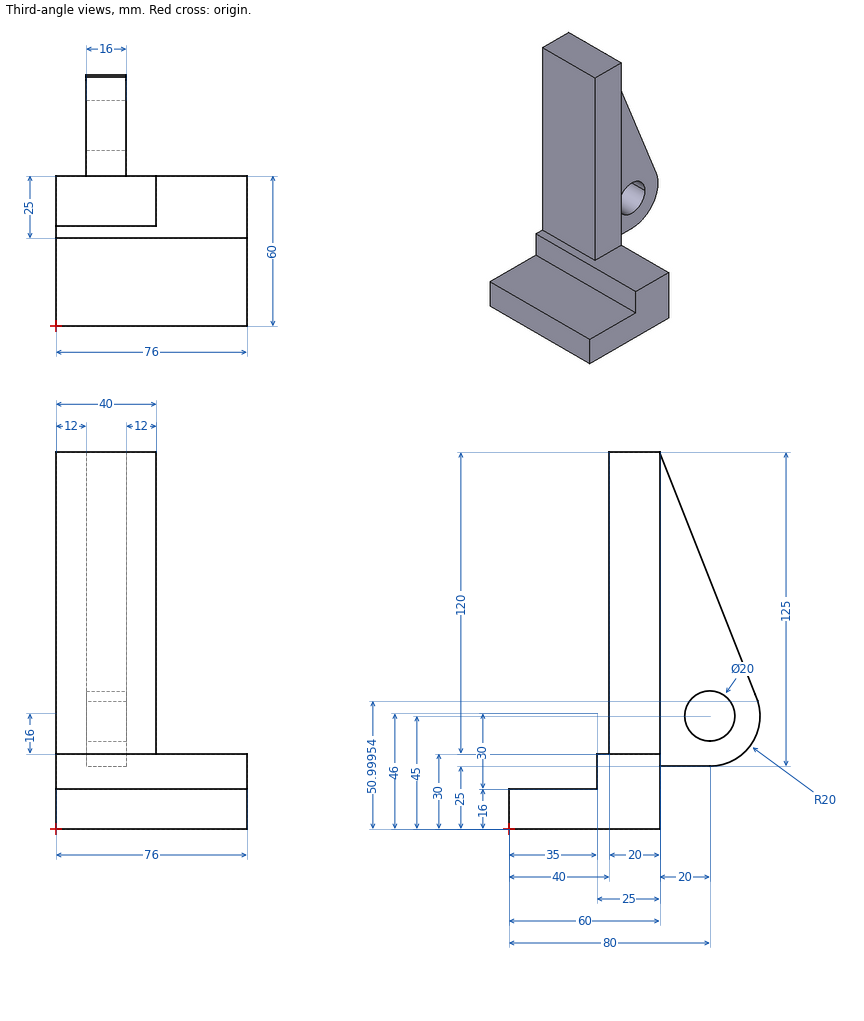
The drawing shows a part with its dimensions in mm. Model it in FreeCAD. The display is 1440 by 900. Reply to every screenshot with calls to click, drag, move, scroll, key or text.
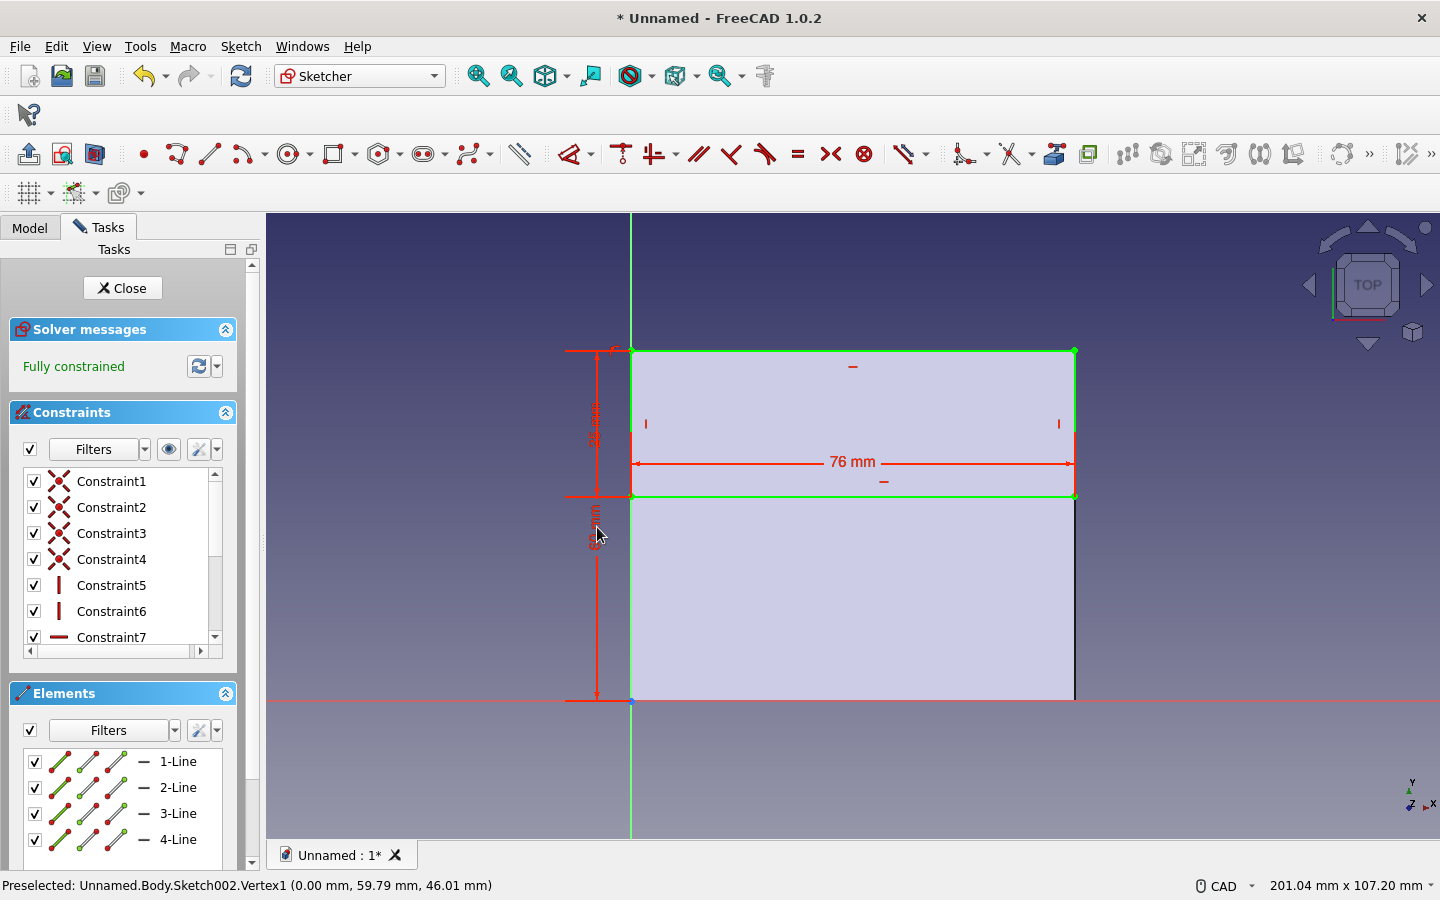
click(123, 288)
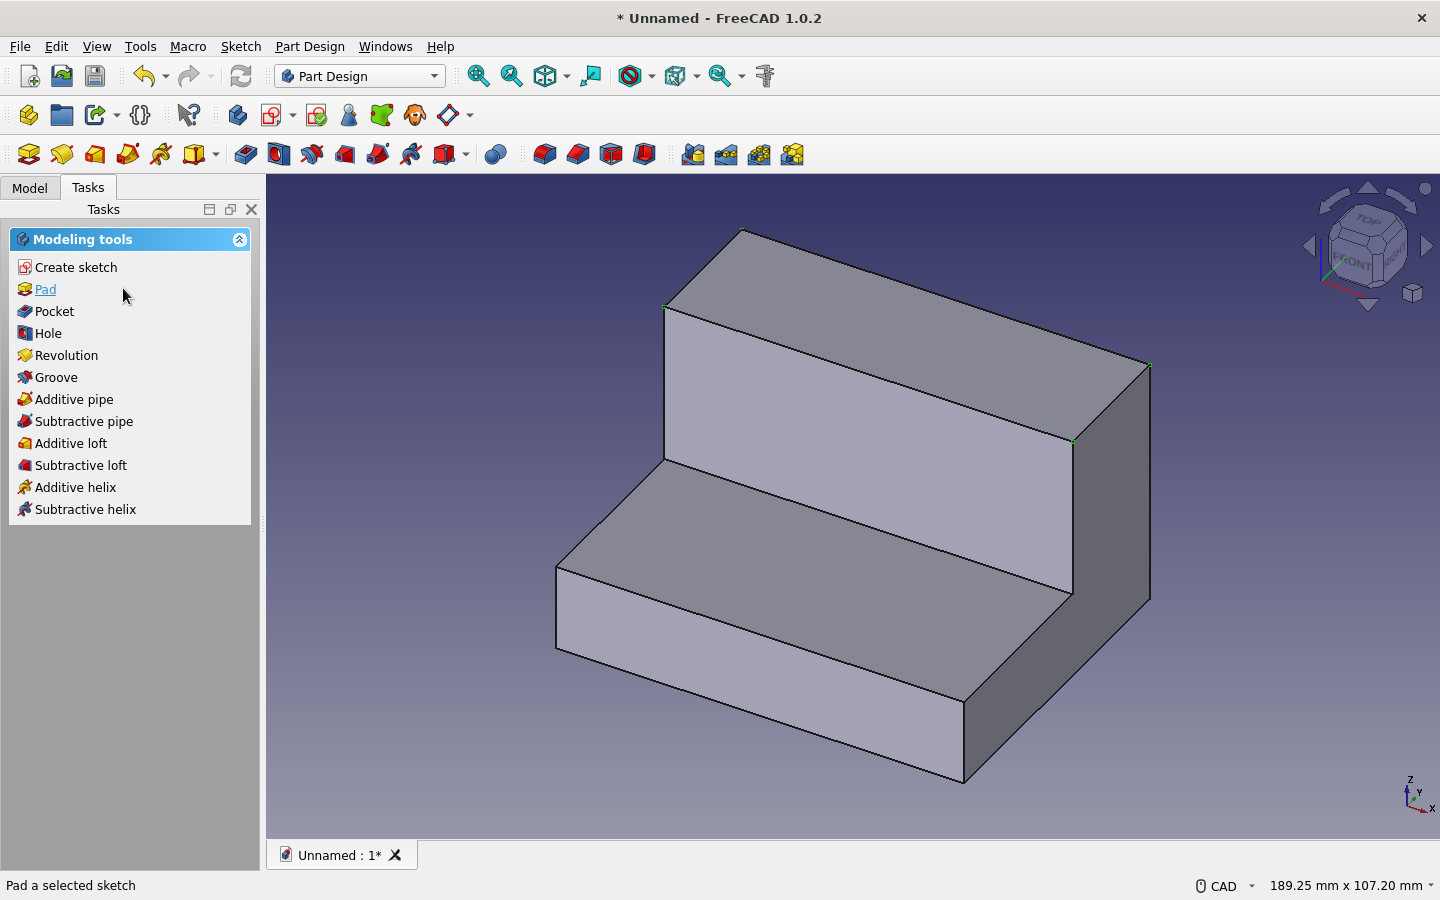
click(246, 154)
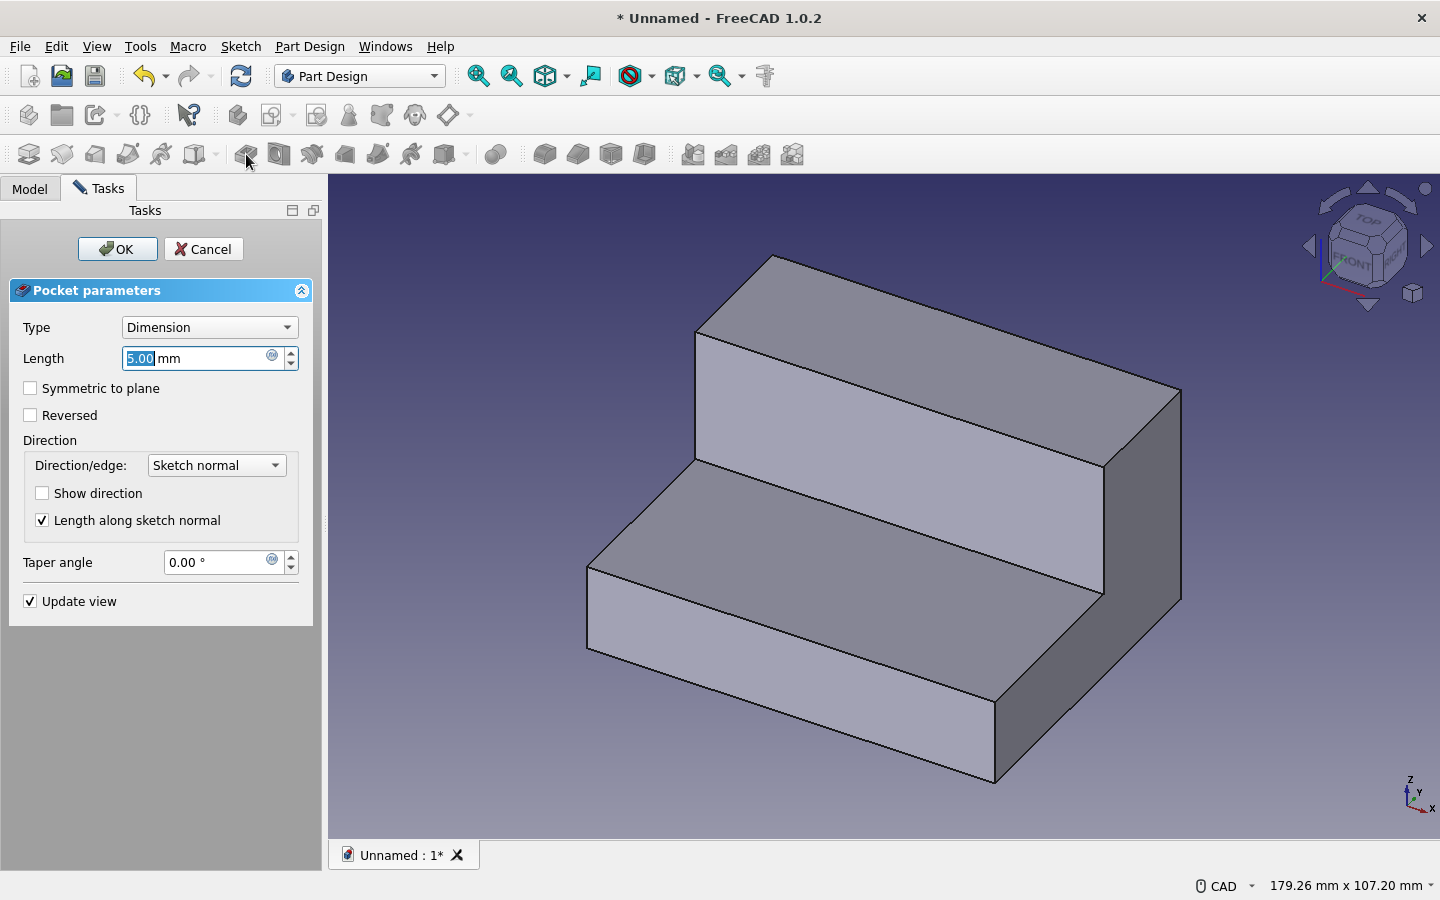
text(16)
key(Tab)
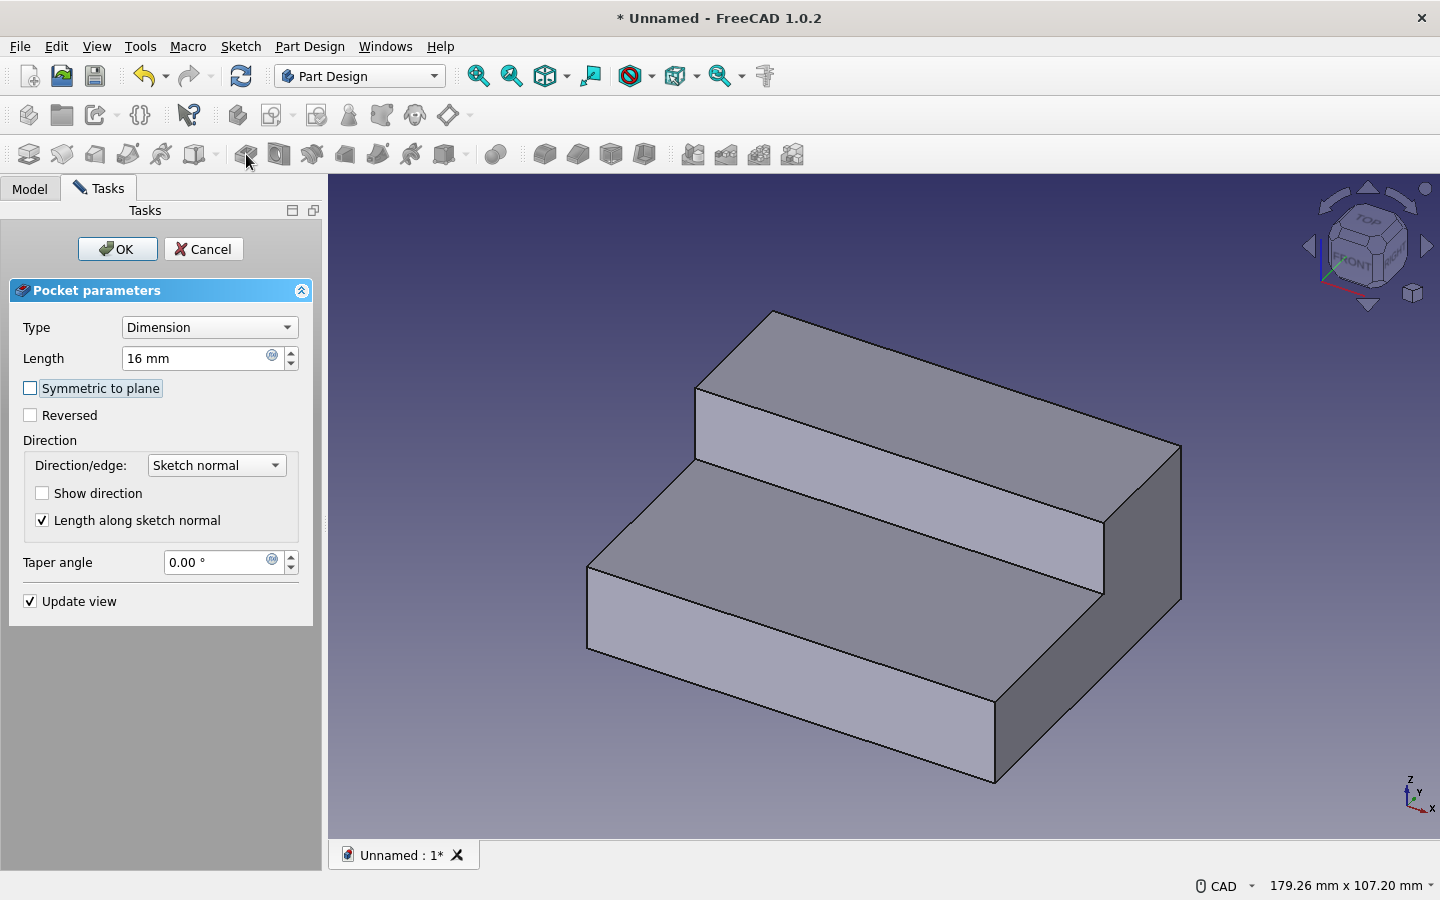
click(118, 249)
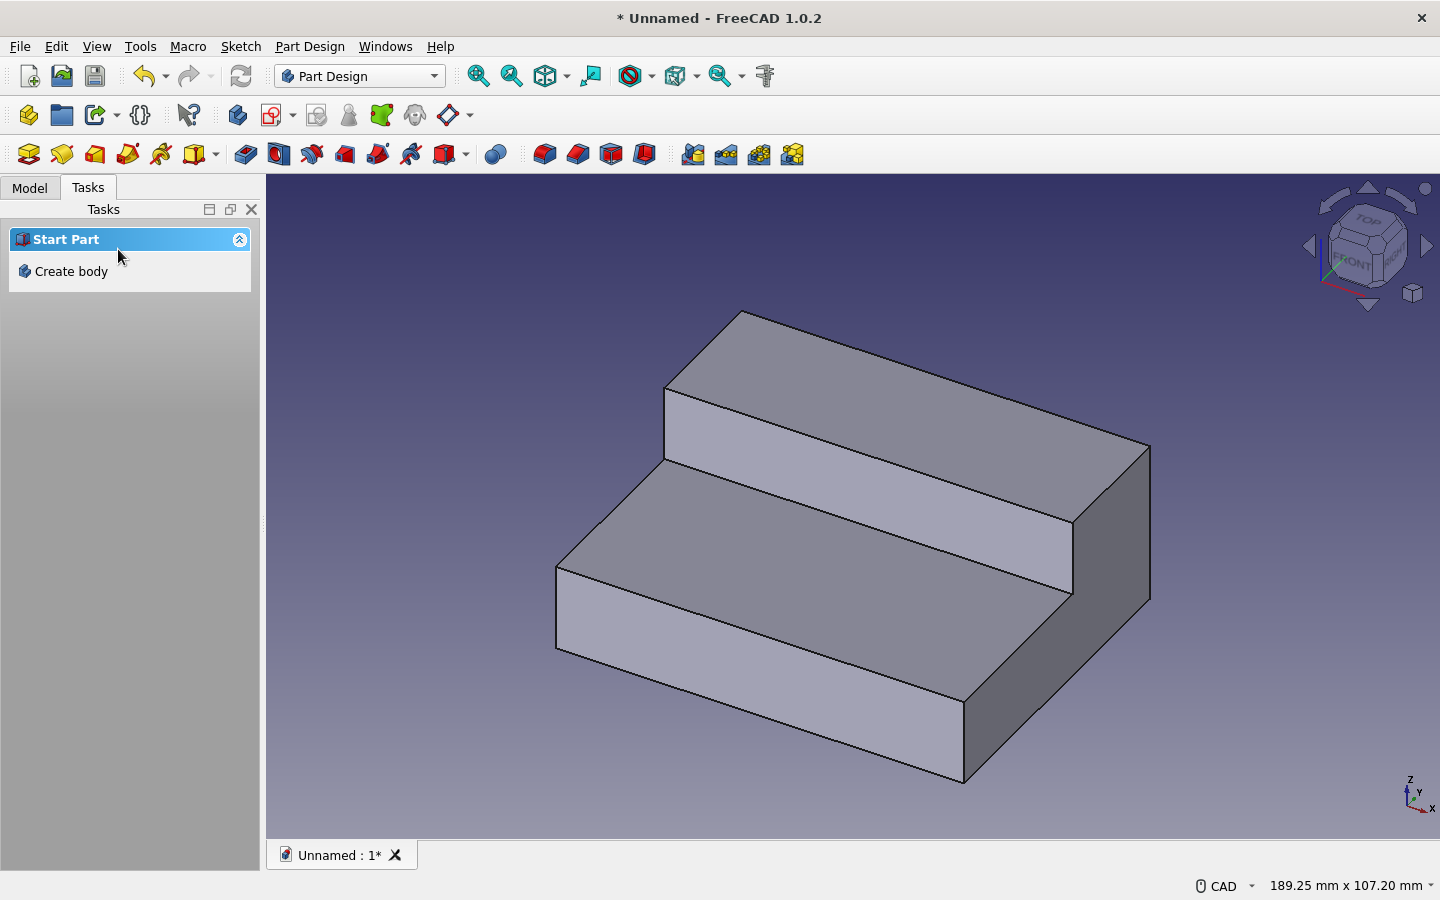
click(270, 116)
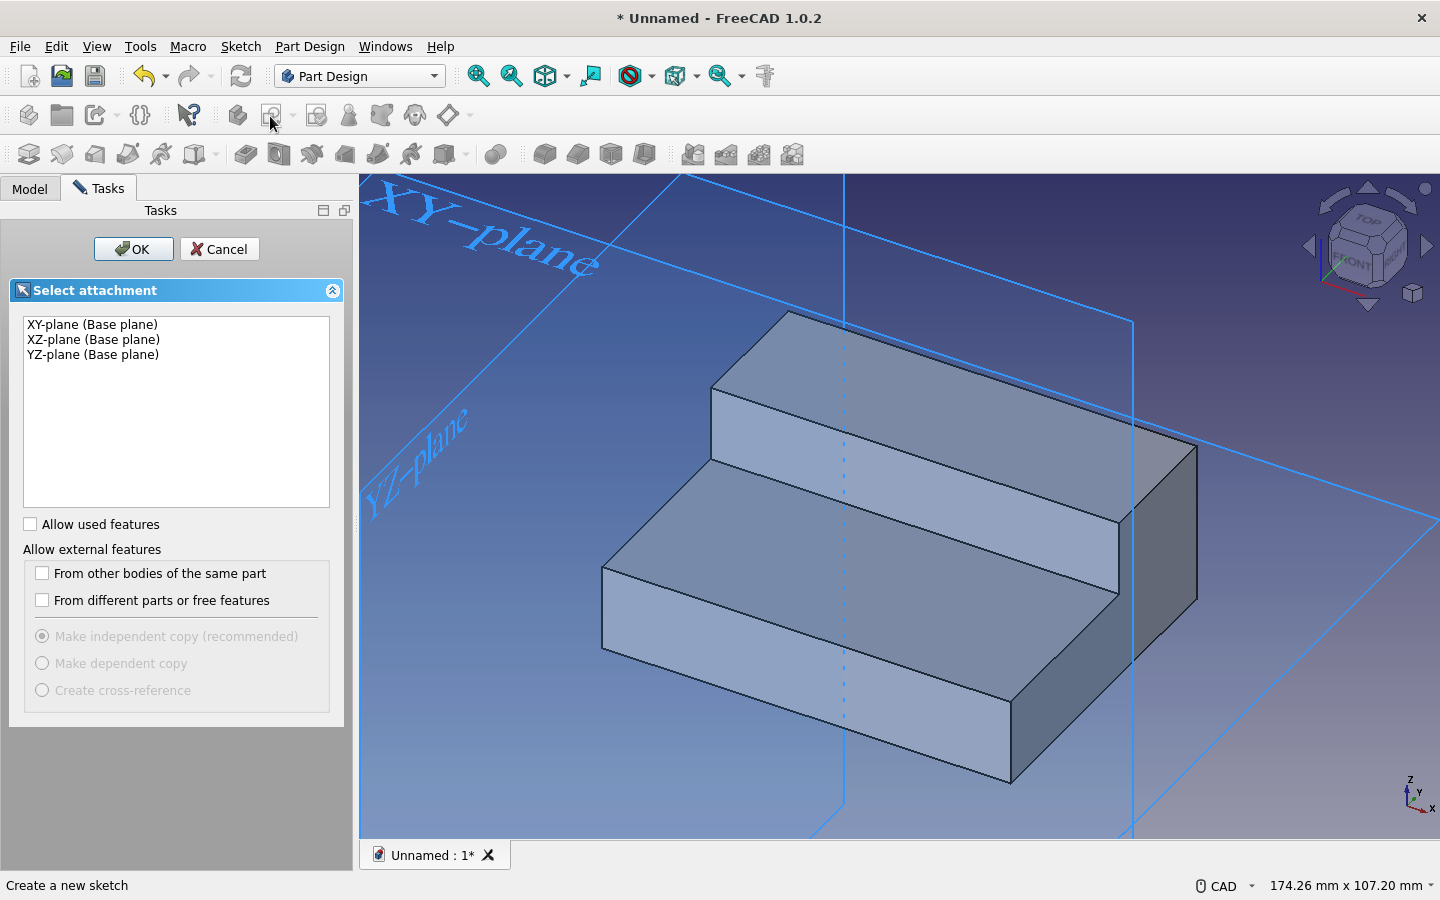
click(84, 354)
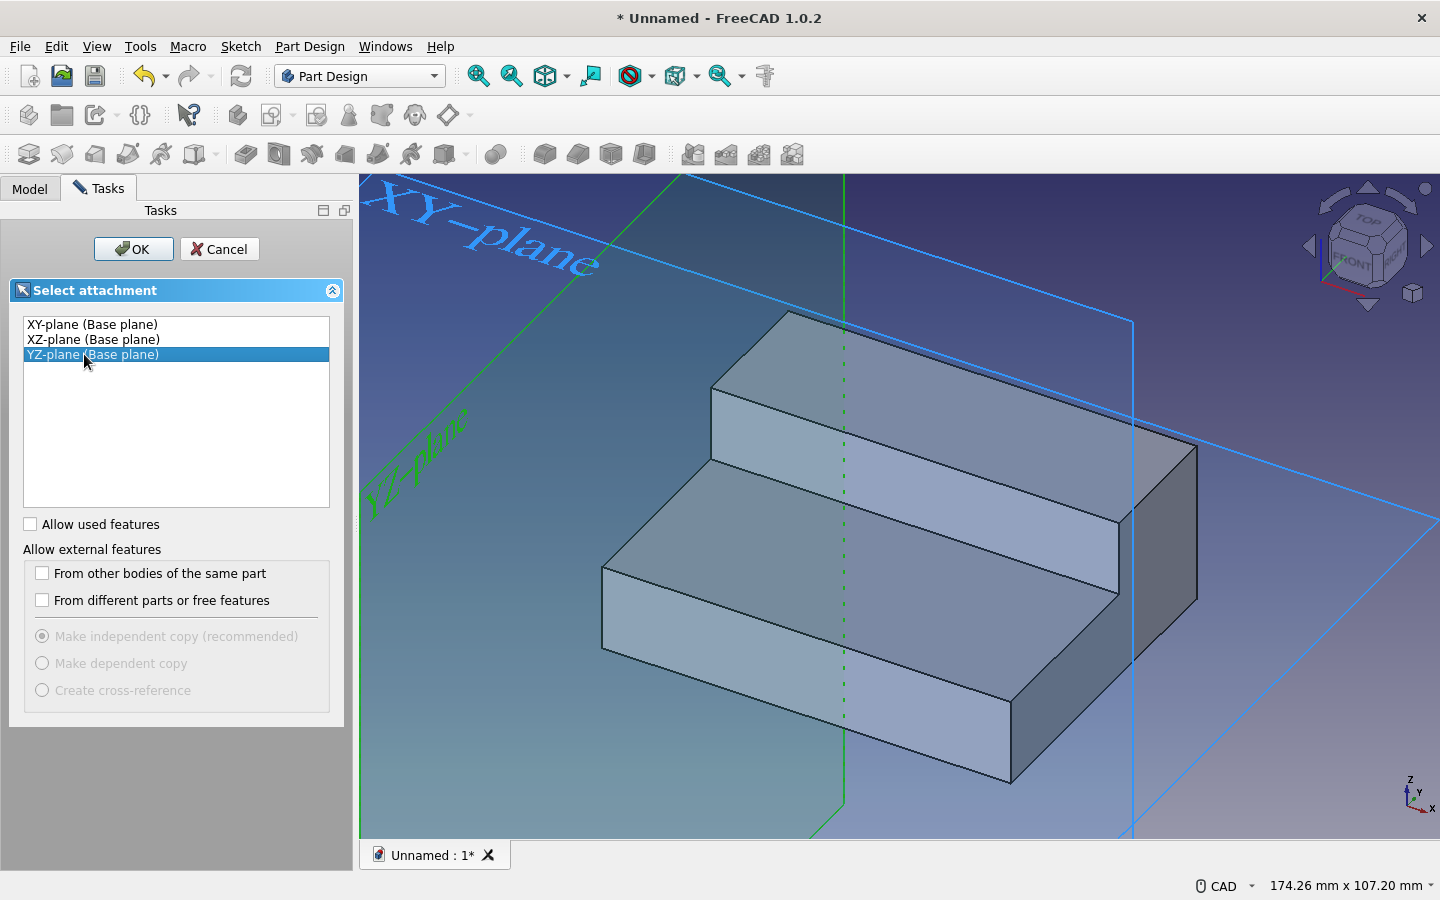
click(134, 249)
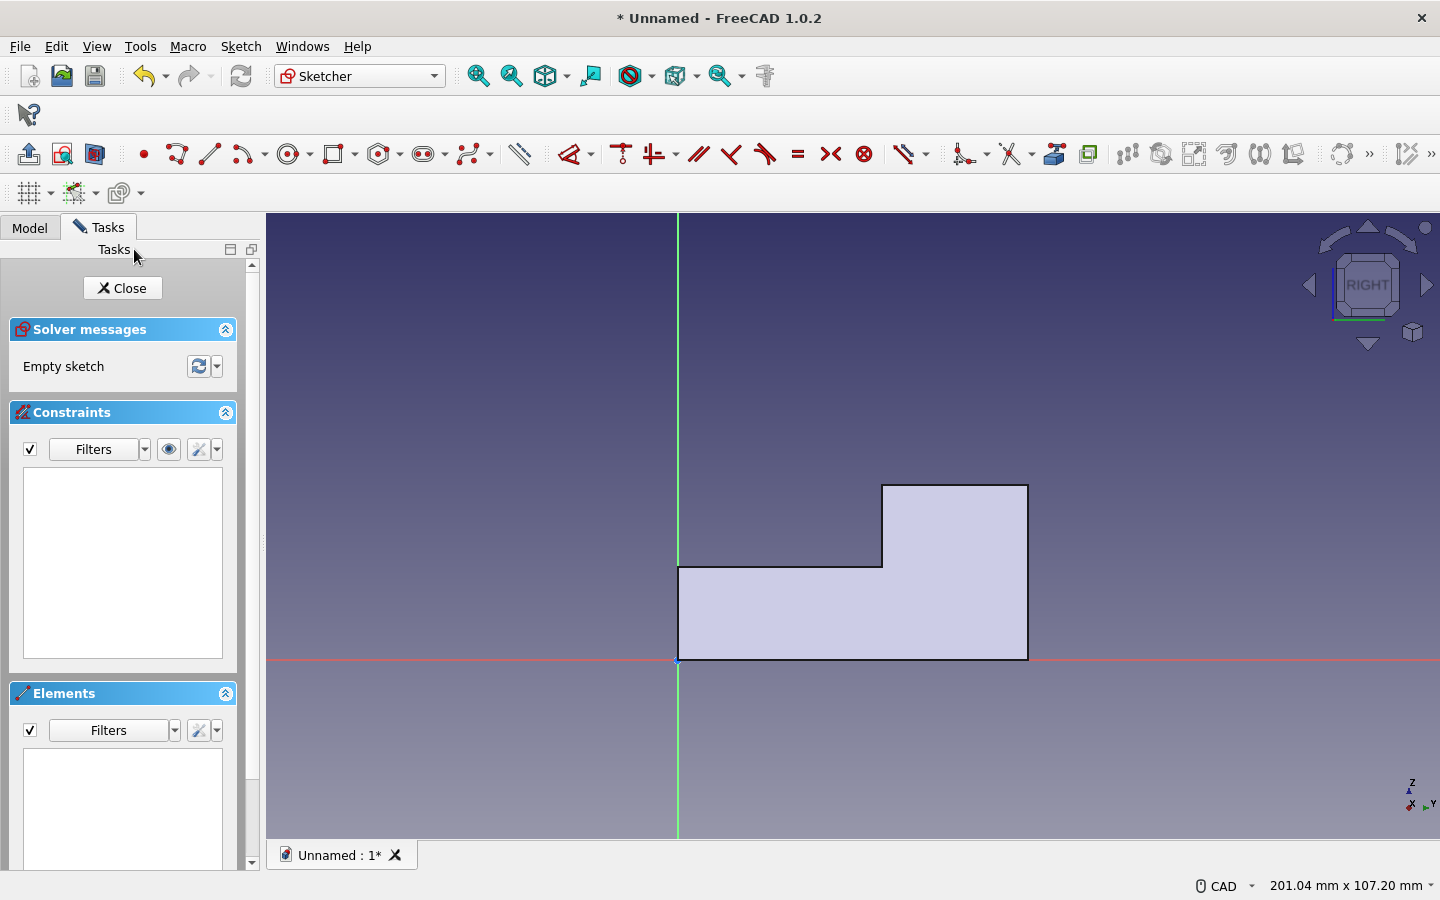
key(q)
key(s)